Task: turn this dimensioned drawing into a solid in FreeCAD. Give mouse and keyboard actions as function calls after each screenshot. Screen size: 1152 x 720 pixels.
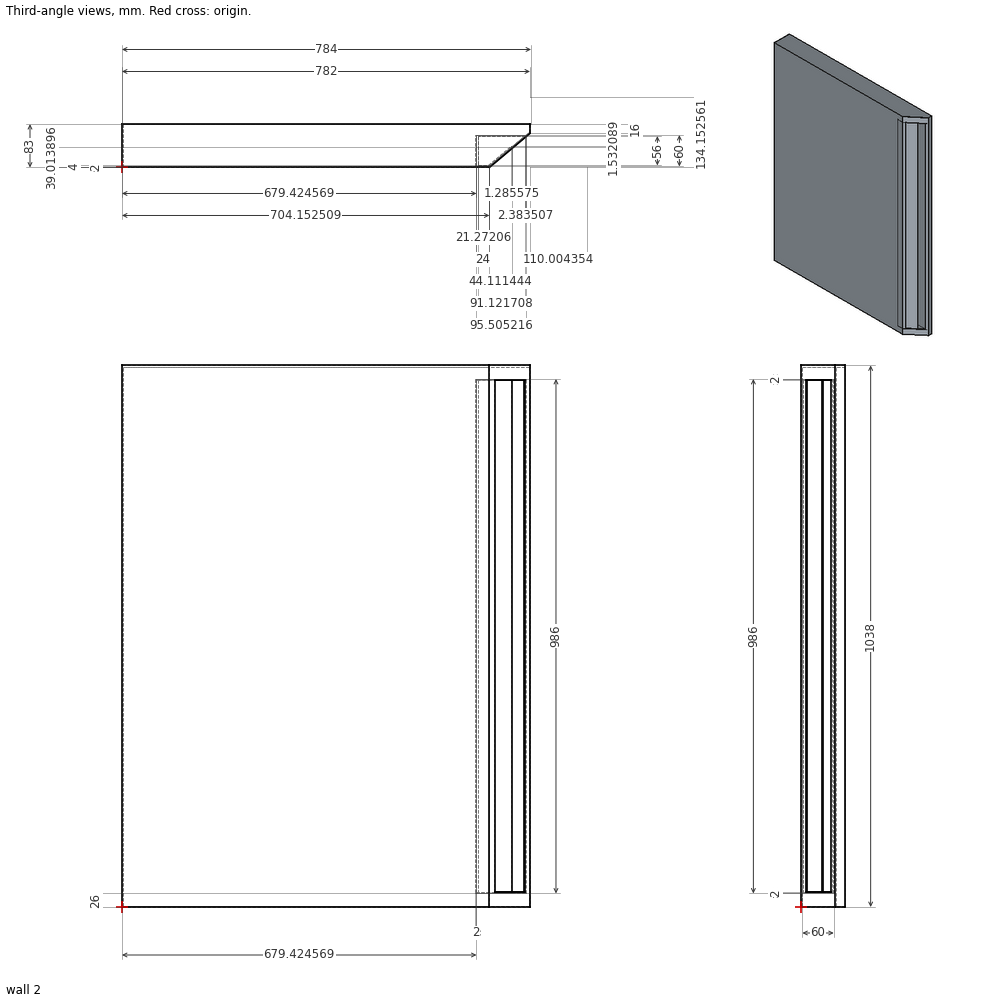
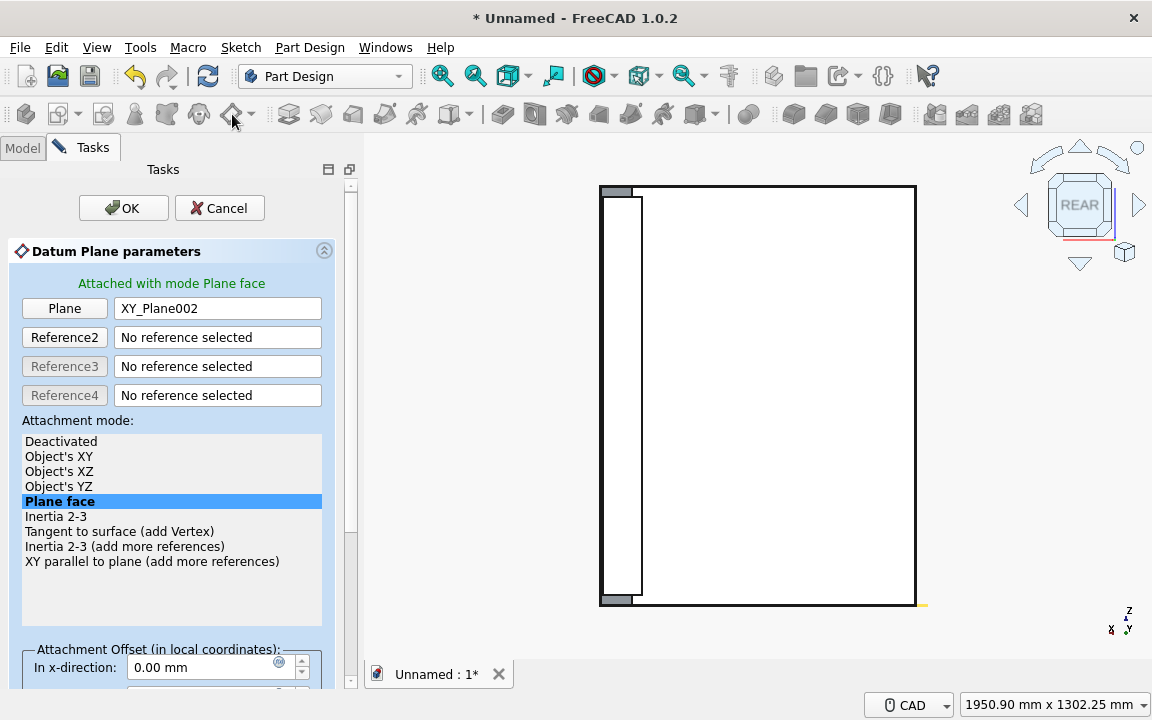
scroll(351, 434, down, 2)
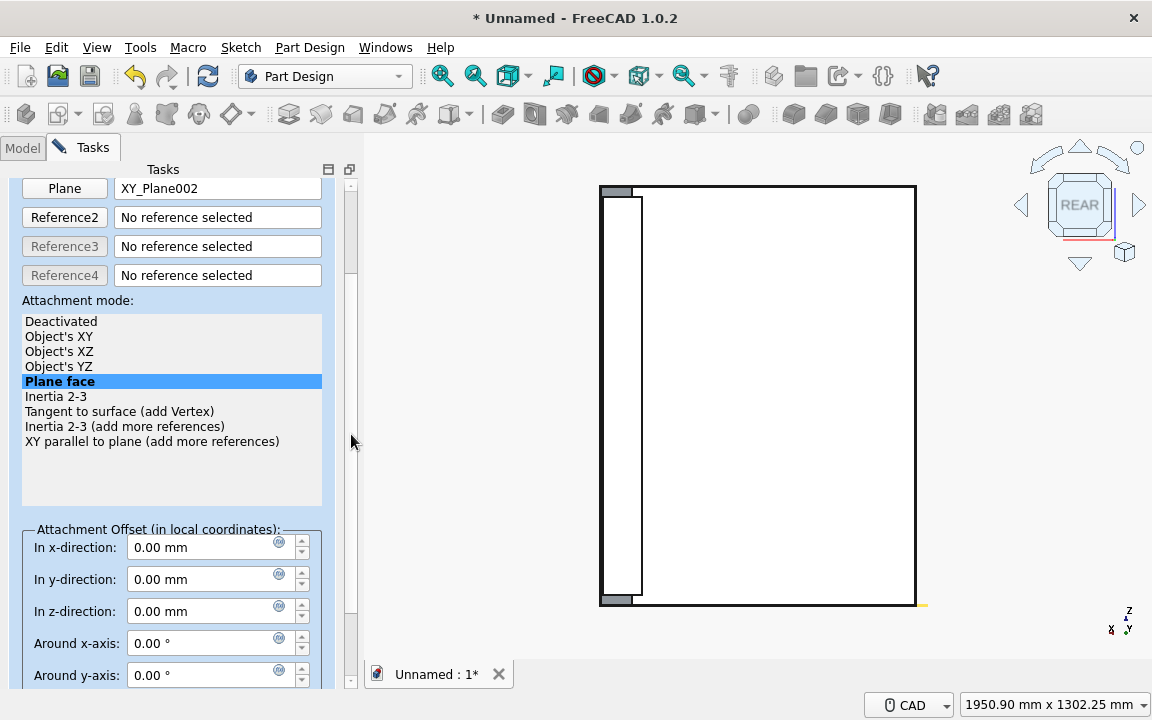
triple_click(210, 611)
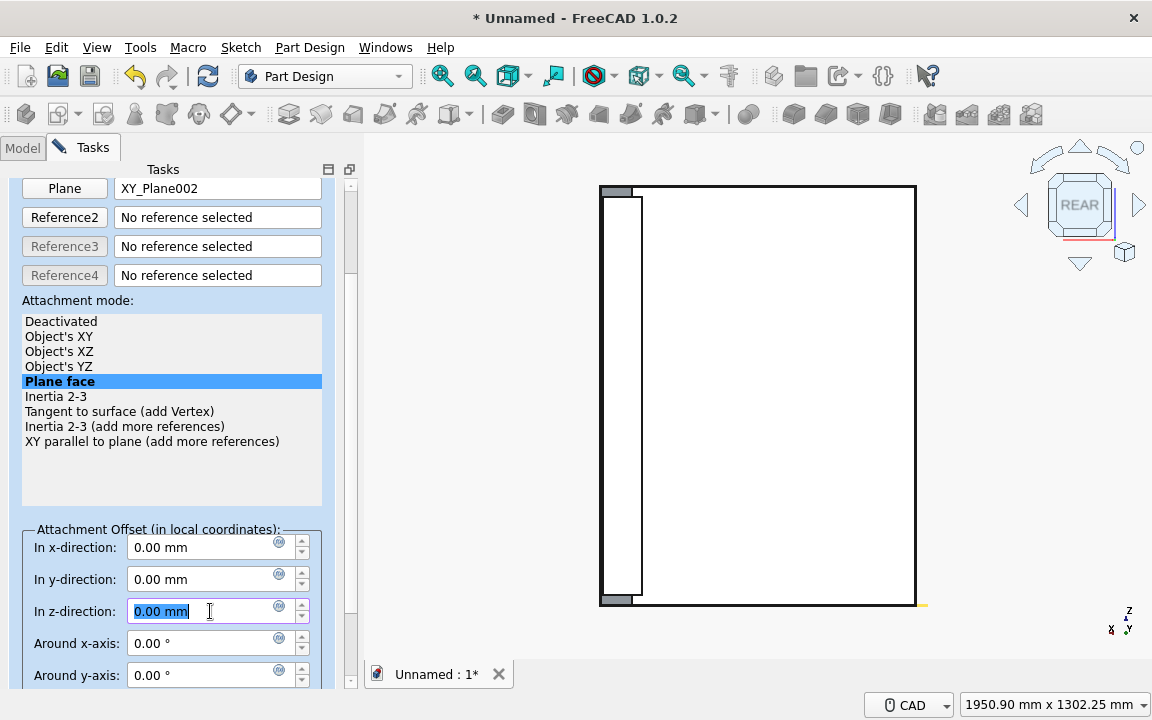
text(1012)
key(Tab)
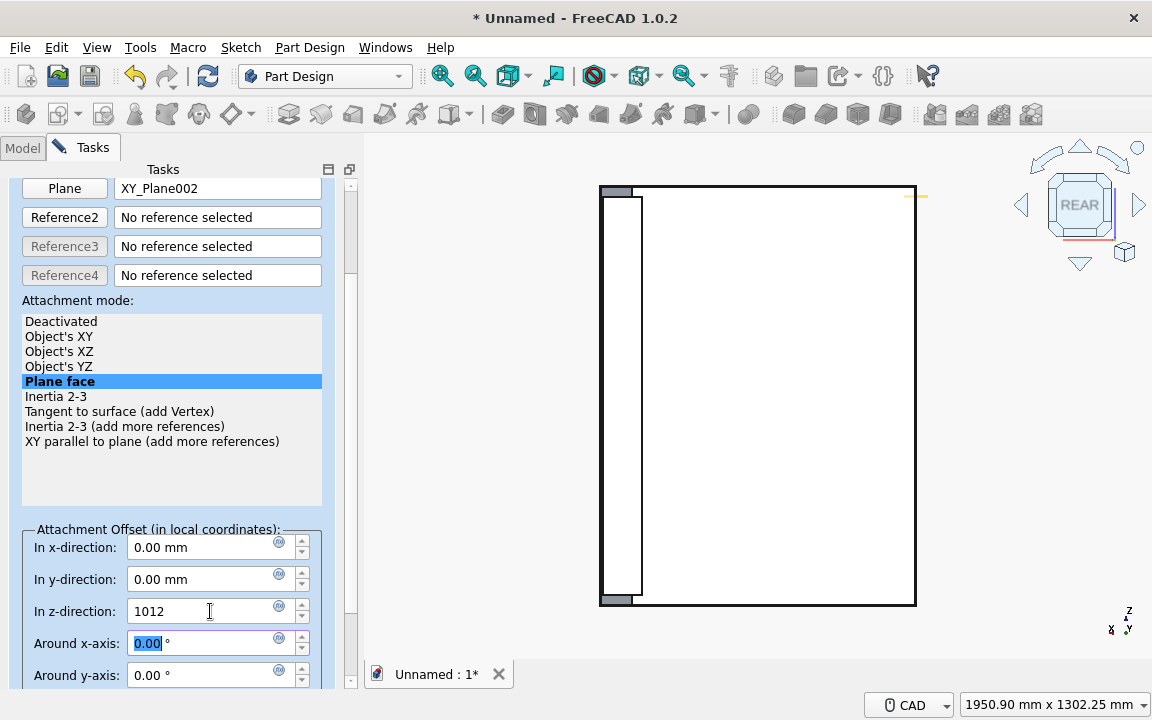
scroll(351, 434, up, 3)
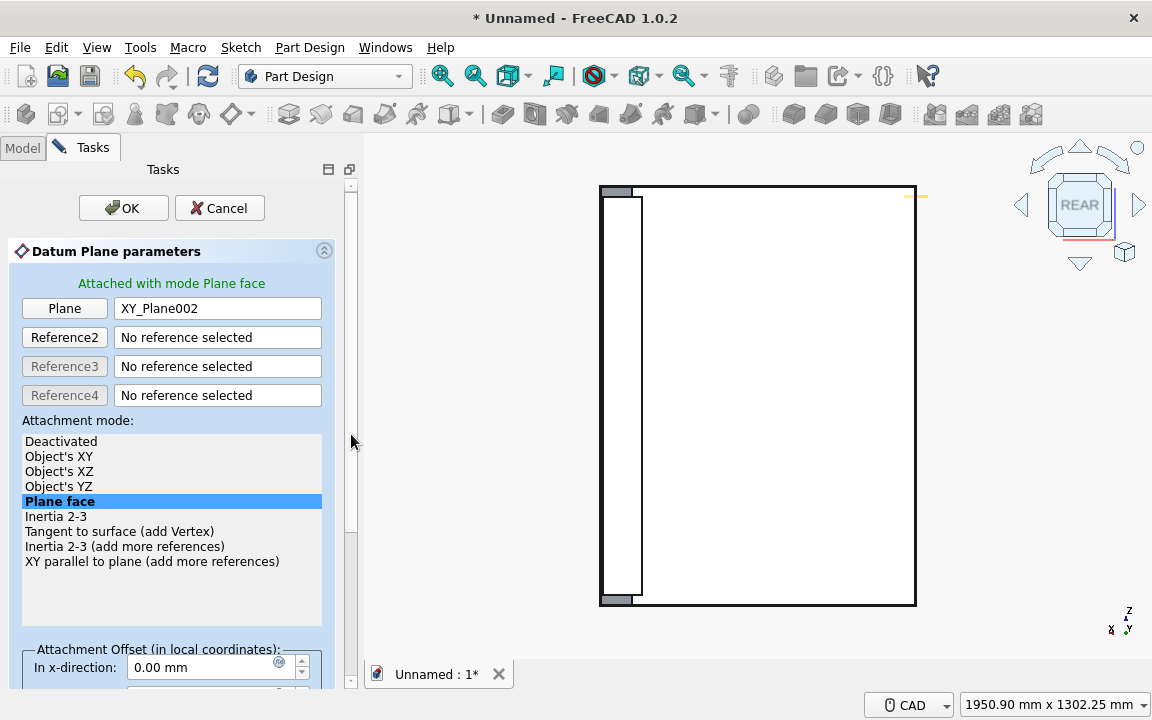
click(124, 208)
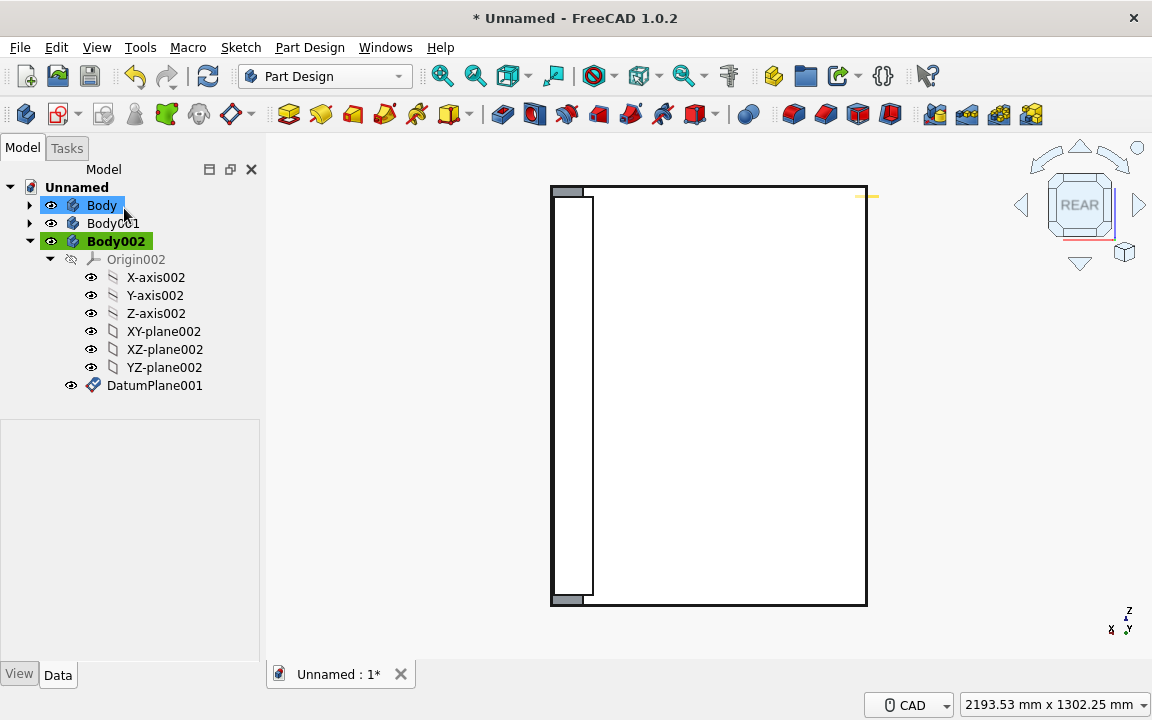
click(116, 385)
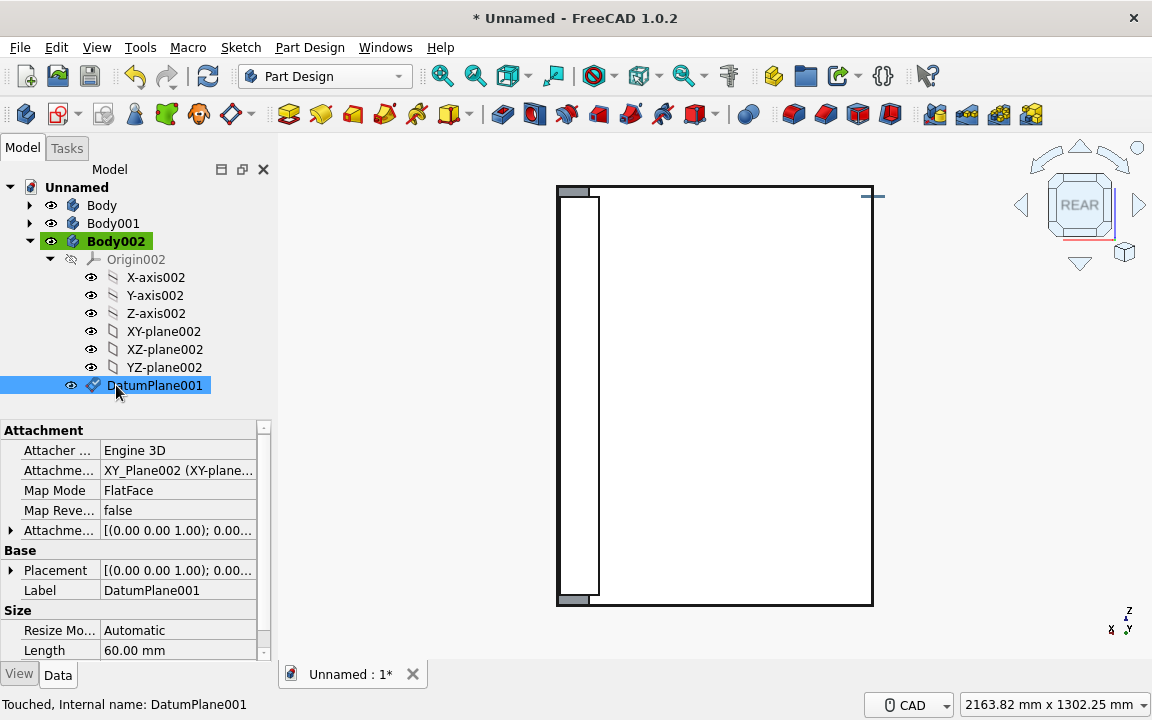
click(58, 114)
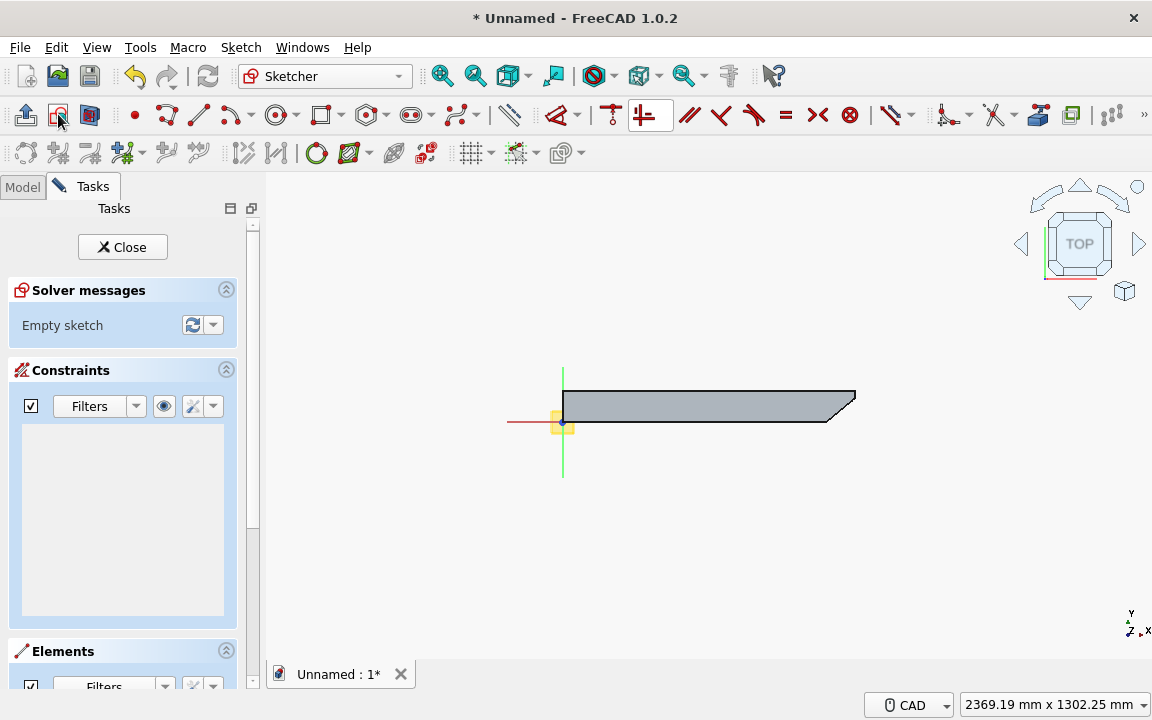
scroll(850, 410, up, 13)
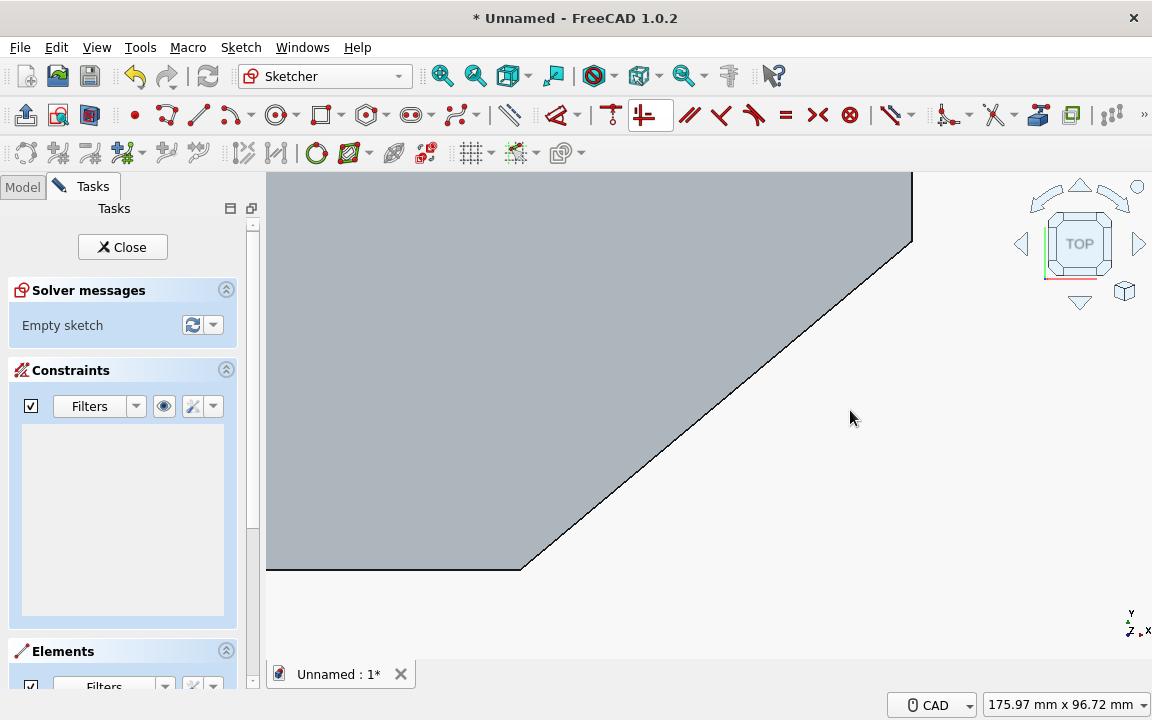
key(g)
key(m)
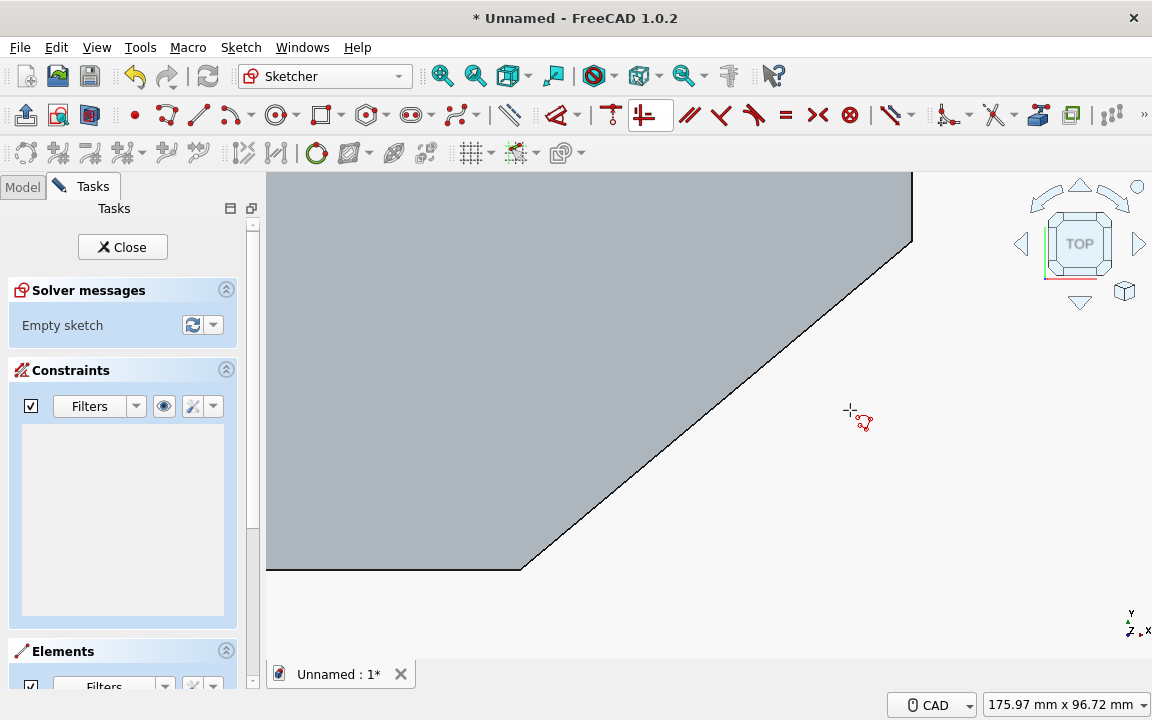
scroll(395, 560, up, 3)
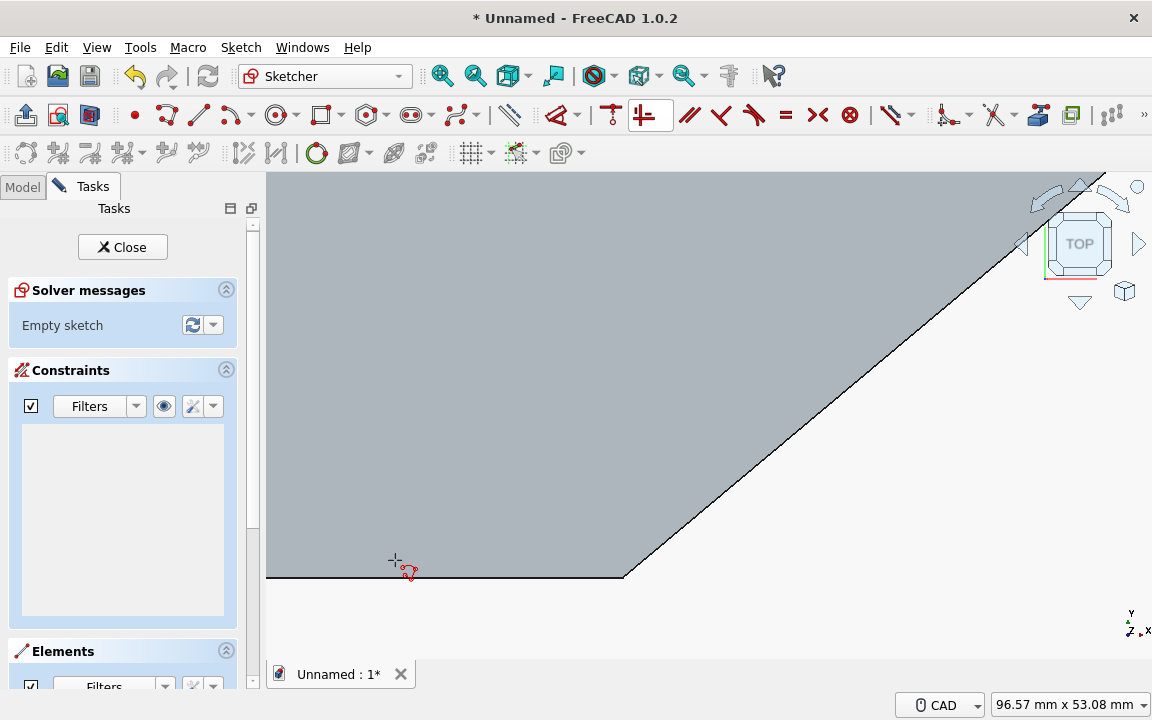
click(396, 559)
click(616, 559)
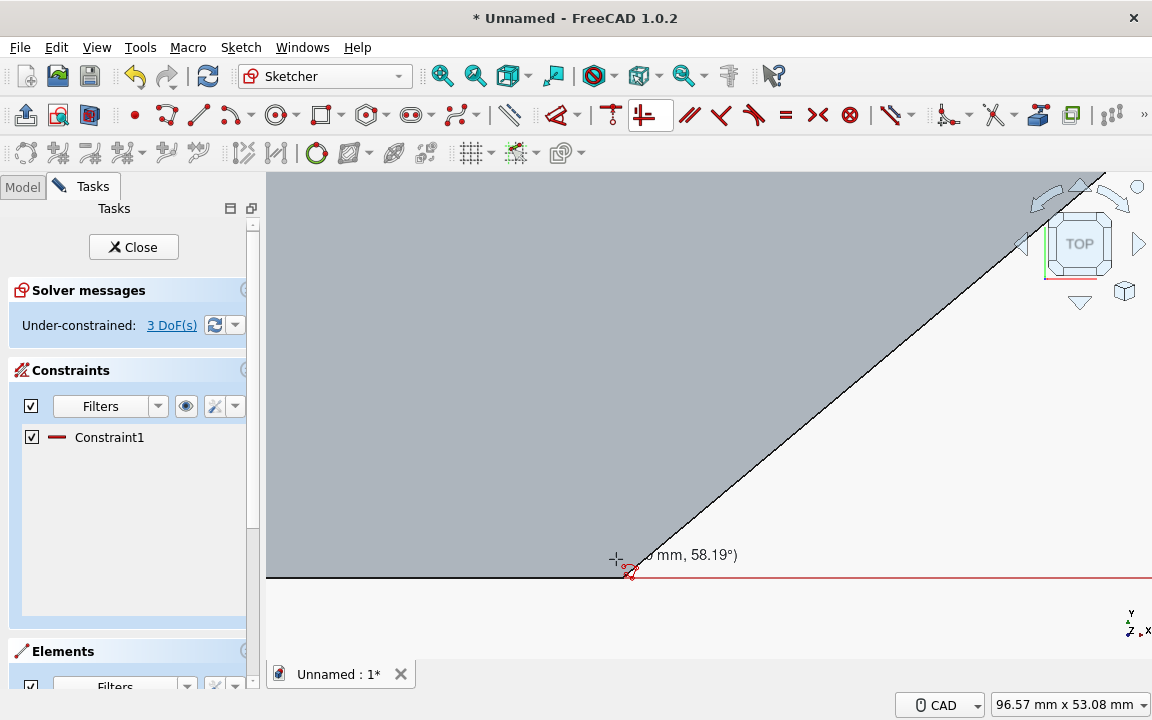
scroll(405, 575, down, 3)